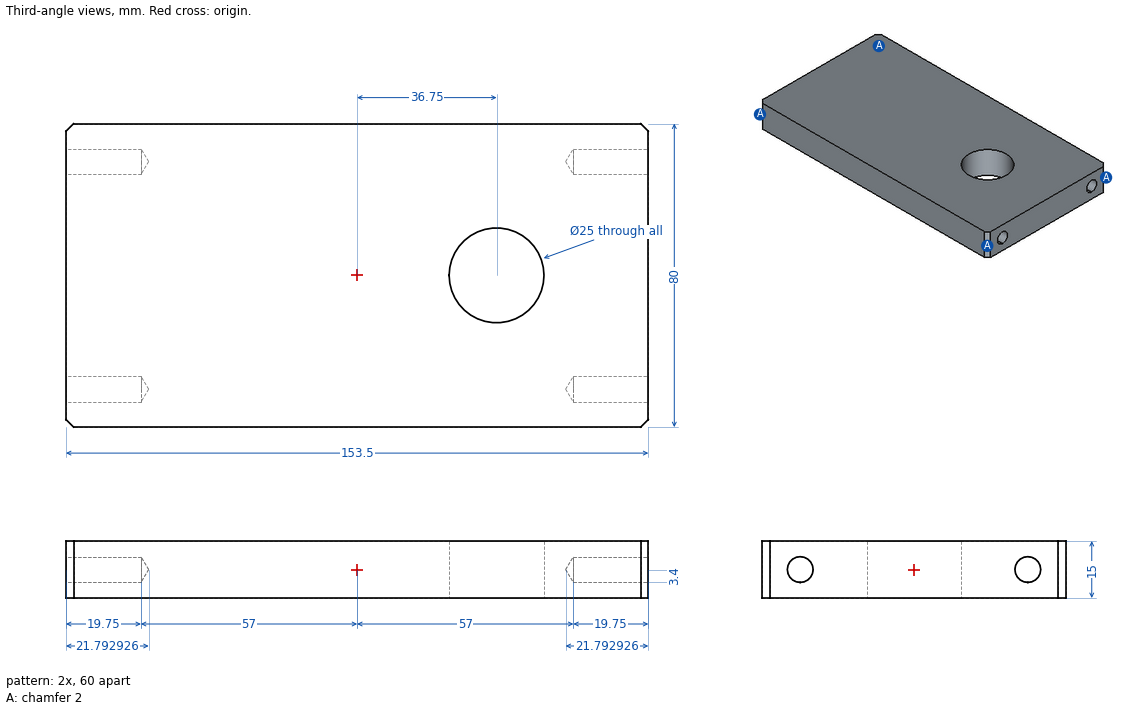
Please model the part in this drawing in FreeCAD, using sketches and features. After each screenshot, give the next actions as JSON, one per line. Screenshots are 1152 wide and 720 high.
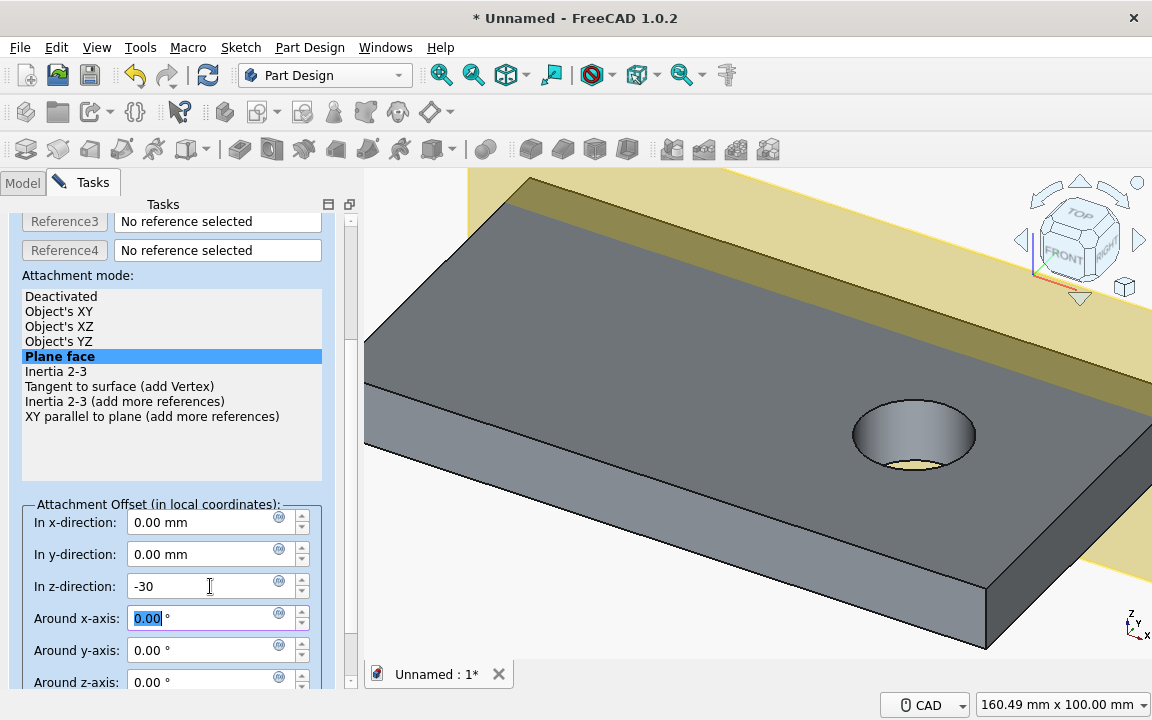
{"action": "scroll", "coordinate": [351, 451], "scroll_direction": "up", "scroll_amount": 4}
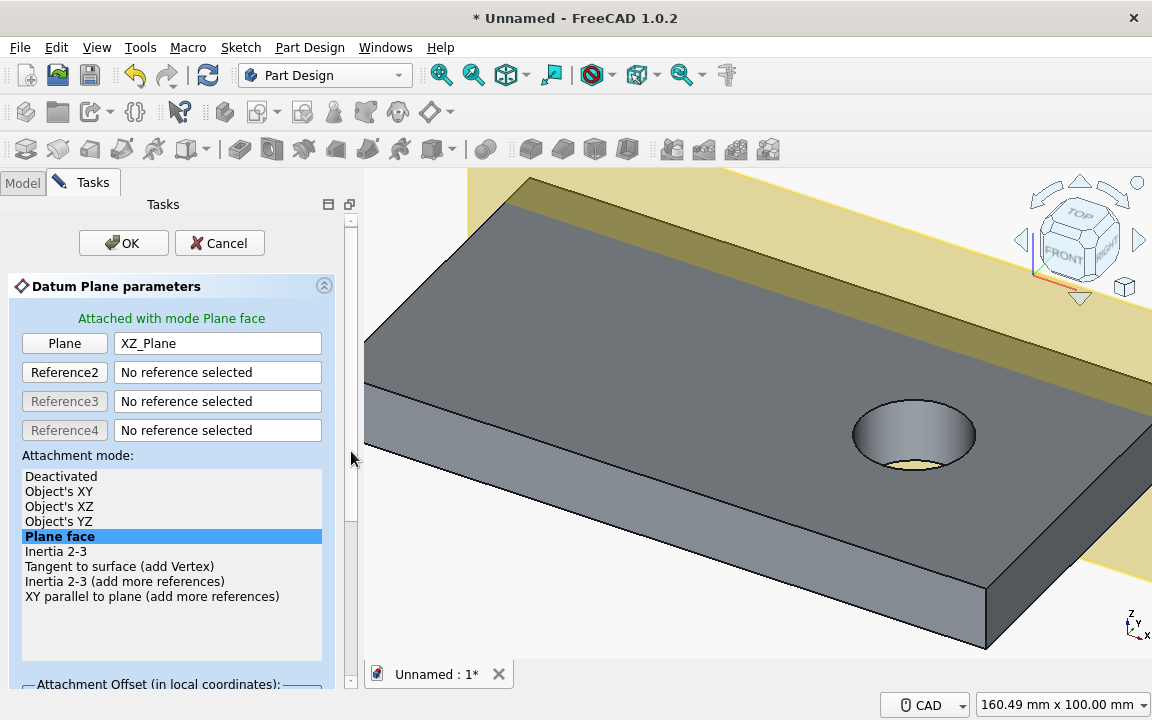
{"action": "left_click", "coordinate": [124, 243]}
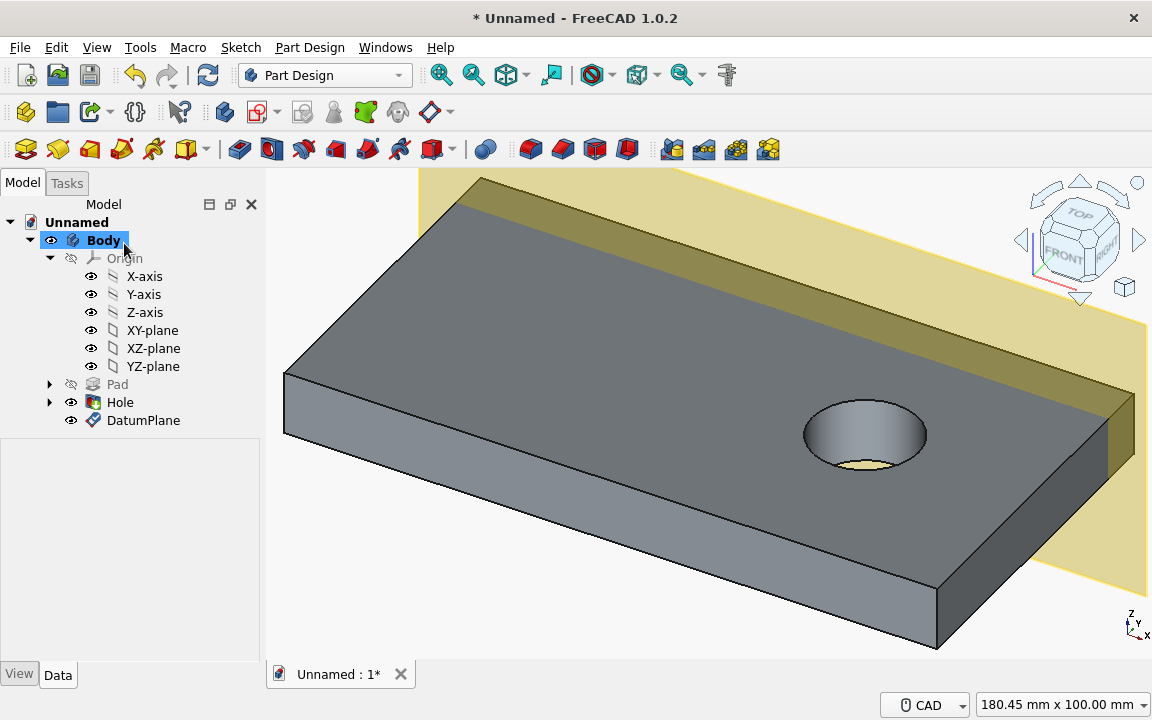
{"action": "left_click", "coordinate": [116, 420]}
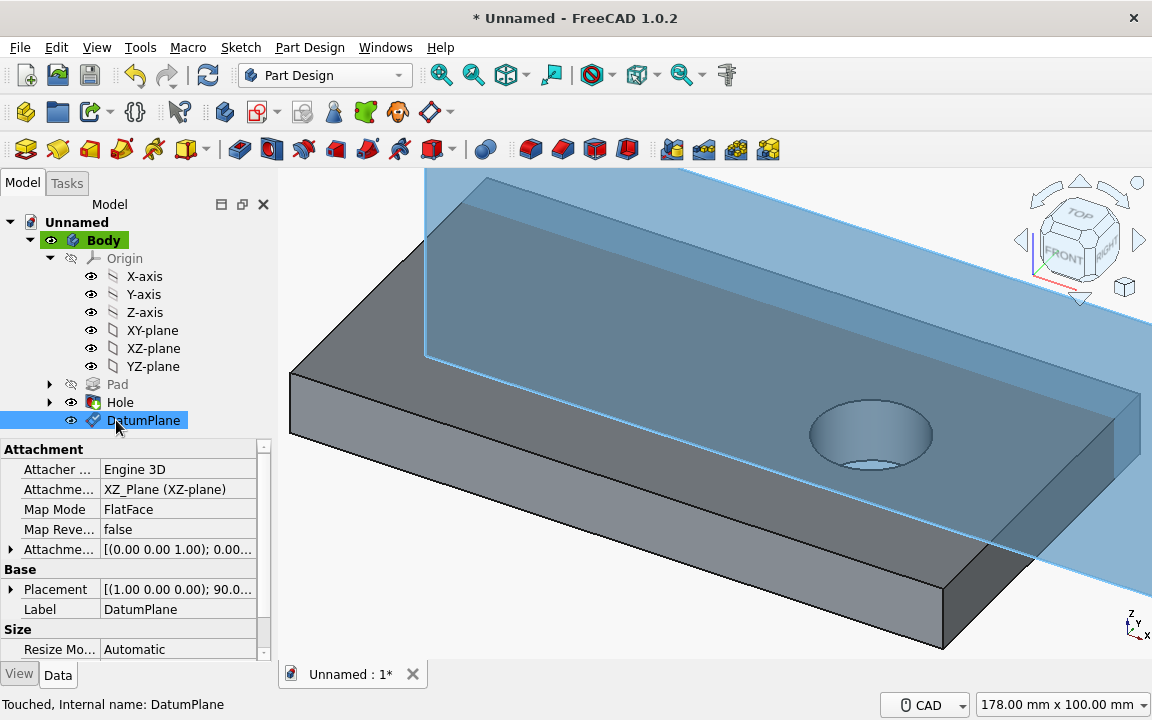
{"action": "left_click", "coordinate": [258, 112]}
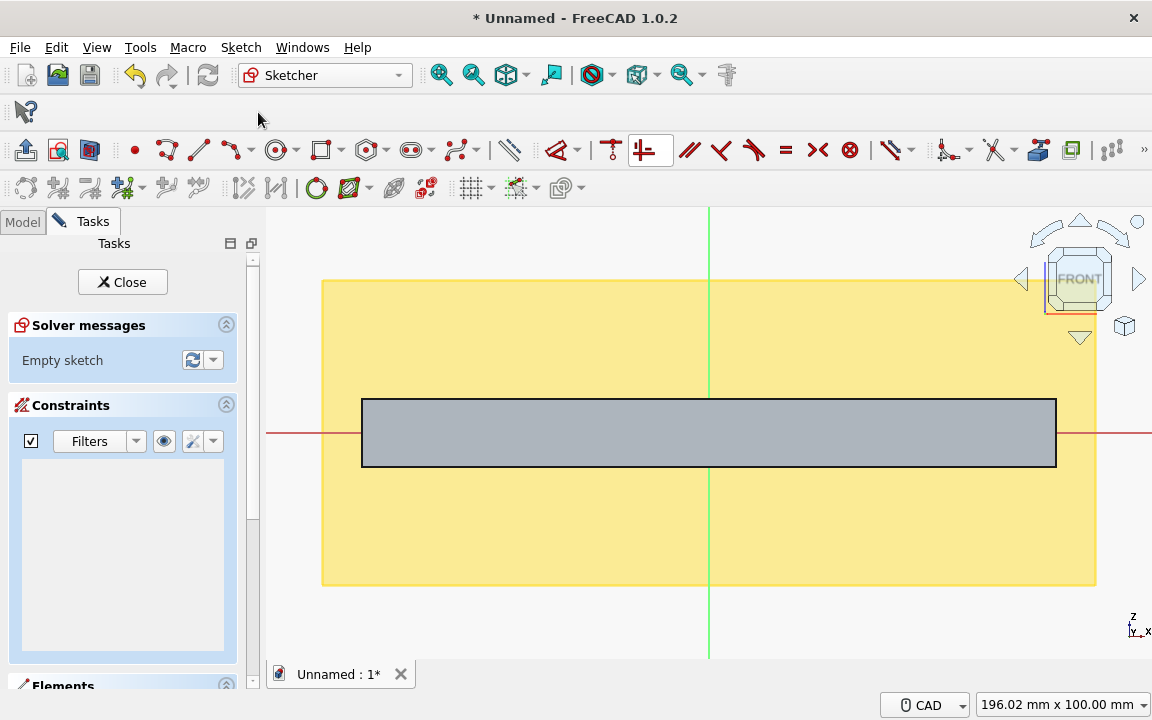
{"action": "left_click", "coordinate": [90, 150]}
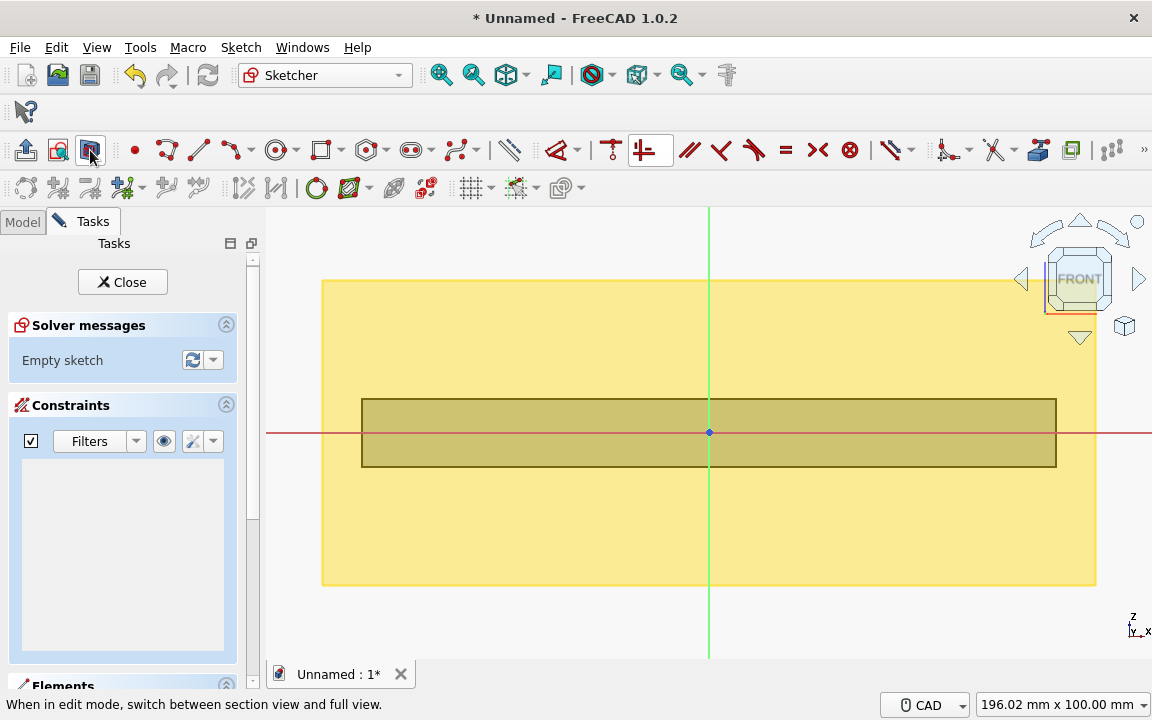
{"action": "scroll", "coordinate": [640, 433], "scroll_direction": "down", "scroll_amount": 5}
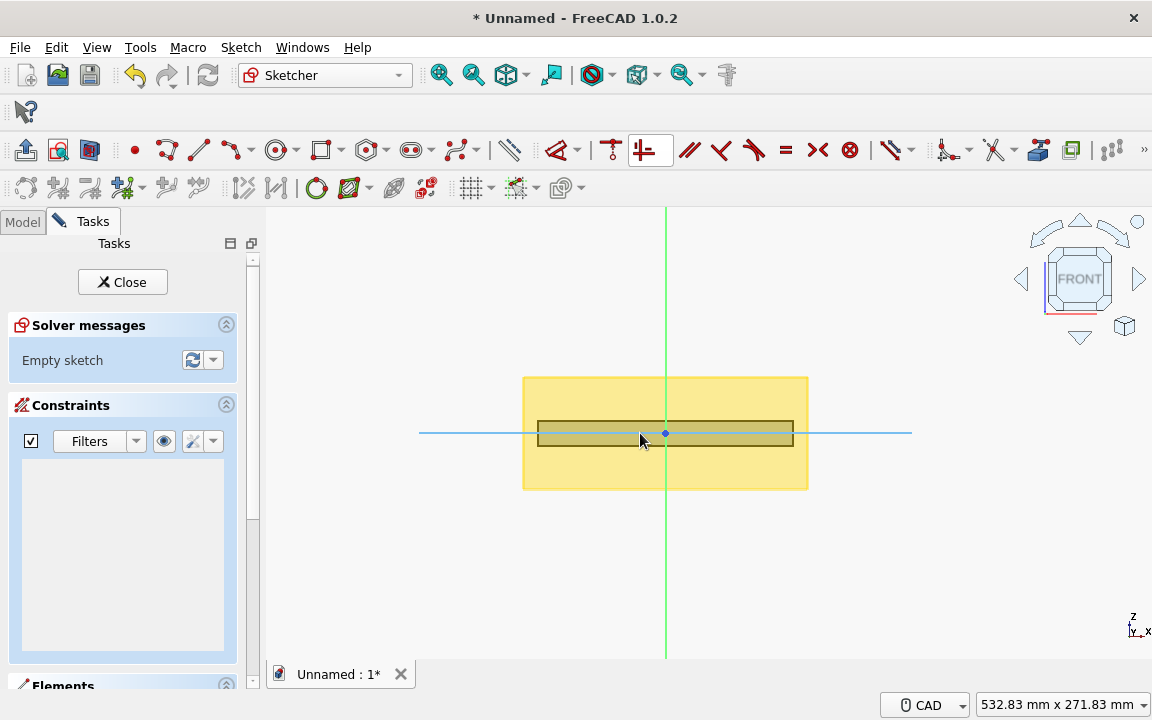
{"action": "scroll", "coordinate": [786, 436], "scroll_direction": "up", "scroll_amount": 13}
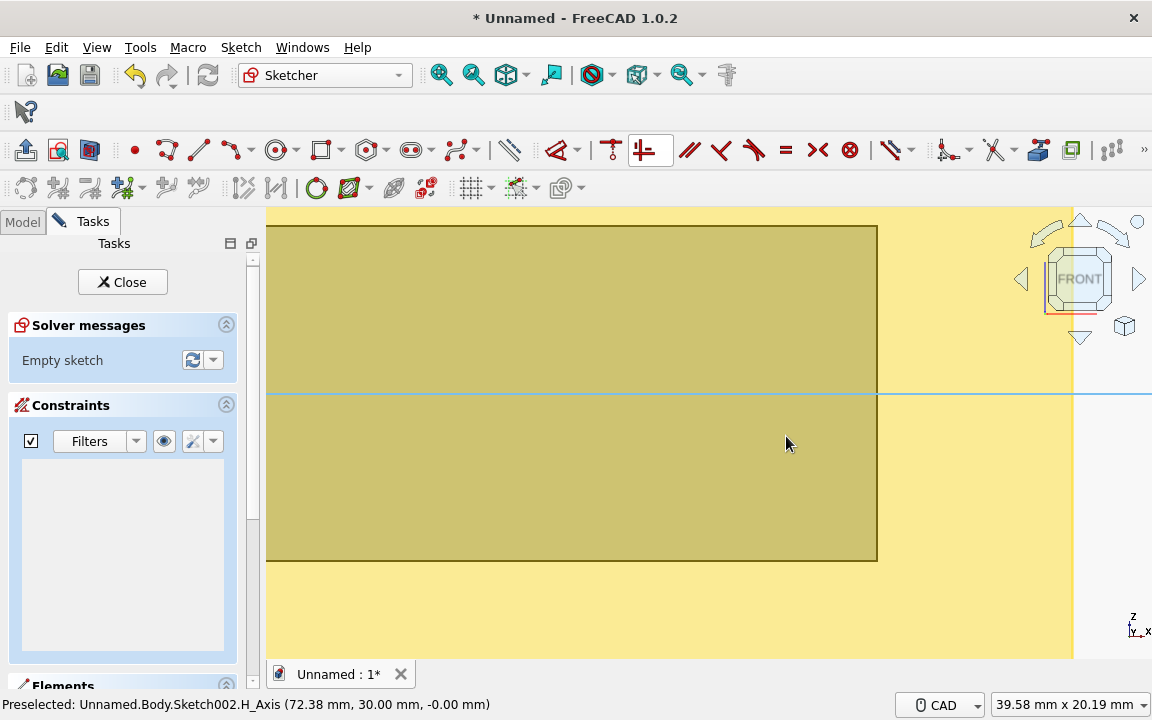
{"action": "key", "text": "g m"}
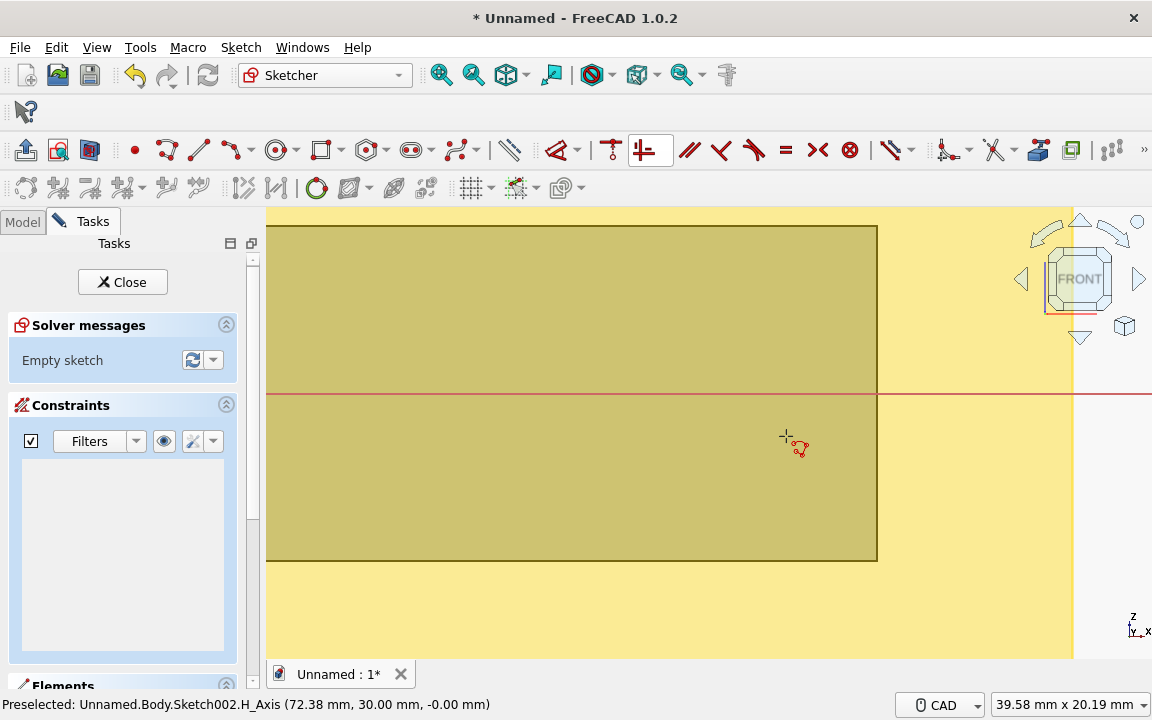
{"action": "left_click", "coordinate": [389, 394]}
{"action": "left_click", "coordinate": [877, 403]}
{"action": "left_click", "coordinate": [877, 470]}
{"action": "left_click", "coordinate": [434, 470]}
{"action": "left_click", "coordinate": [389, 394]}
{"action": "key", "text": "Escape"}
{"action": "key", "text": "Escape"}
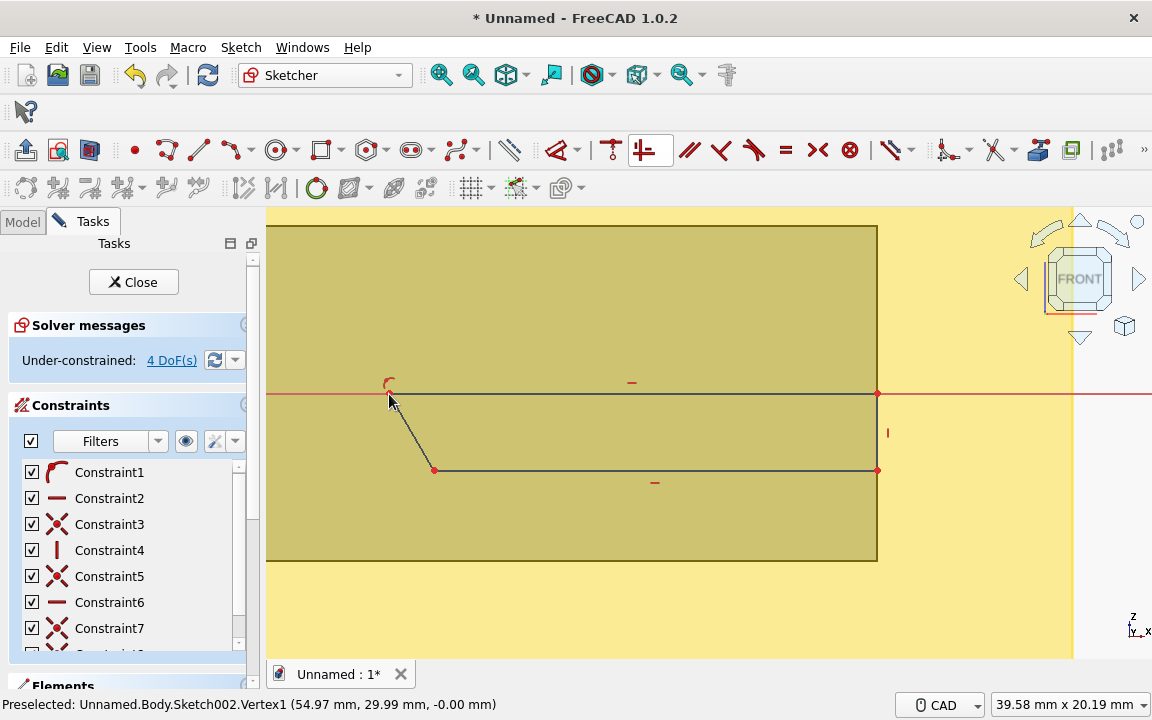
{"action": "key", "text": "d"}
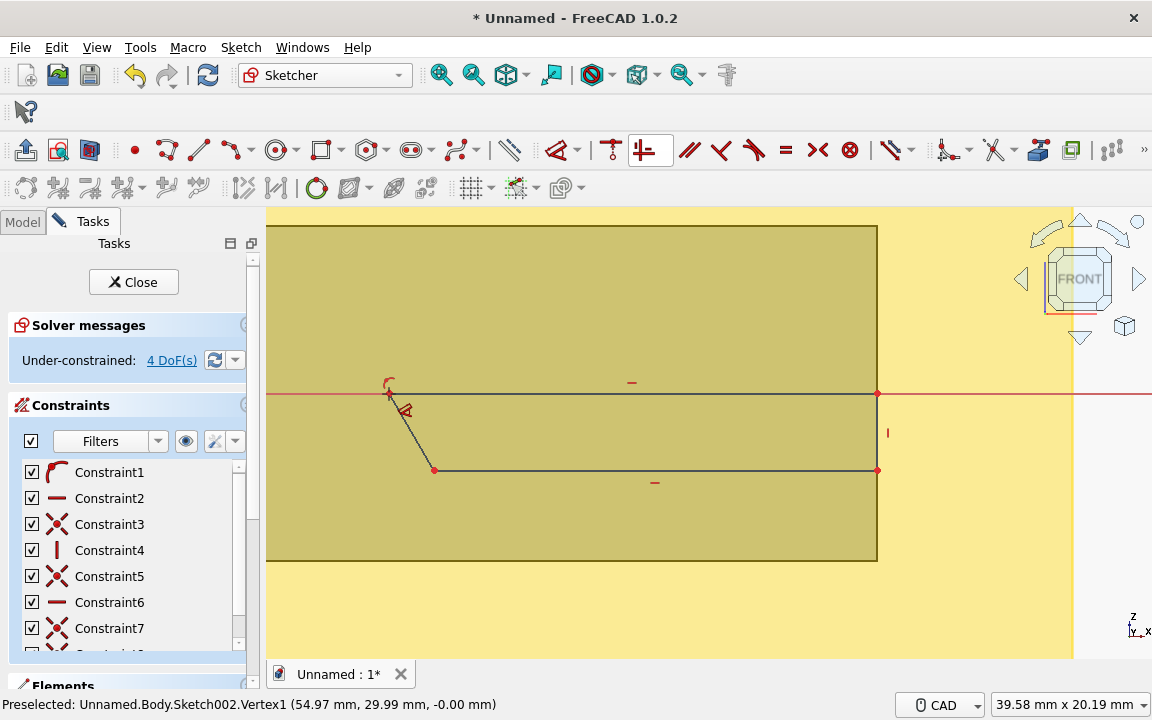
{"action": "left_click", "coordinate": [877, 417]}
{"action": "left_click", "coordinate": [911, 432]}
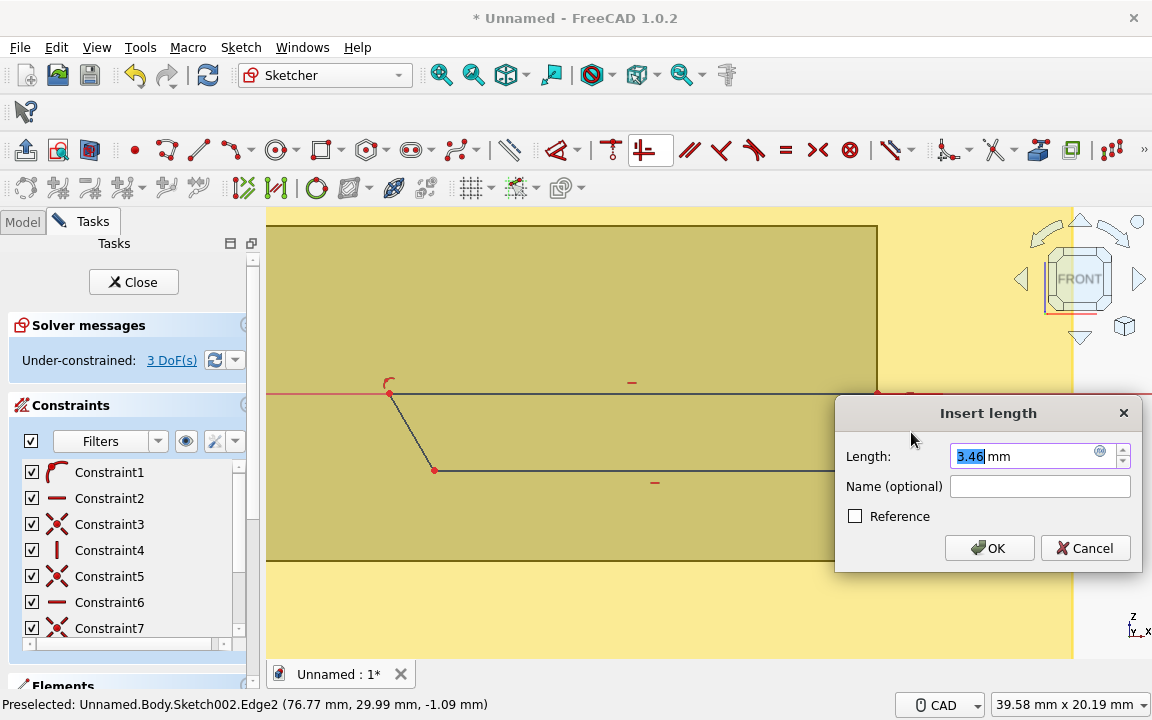
{"action": "type", "text": "3.4"}
{"action": "key", "text": "Return"}